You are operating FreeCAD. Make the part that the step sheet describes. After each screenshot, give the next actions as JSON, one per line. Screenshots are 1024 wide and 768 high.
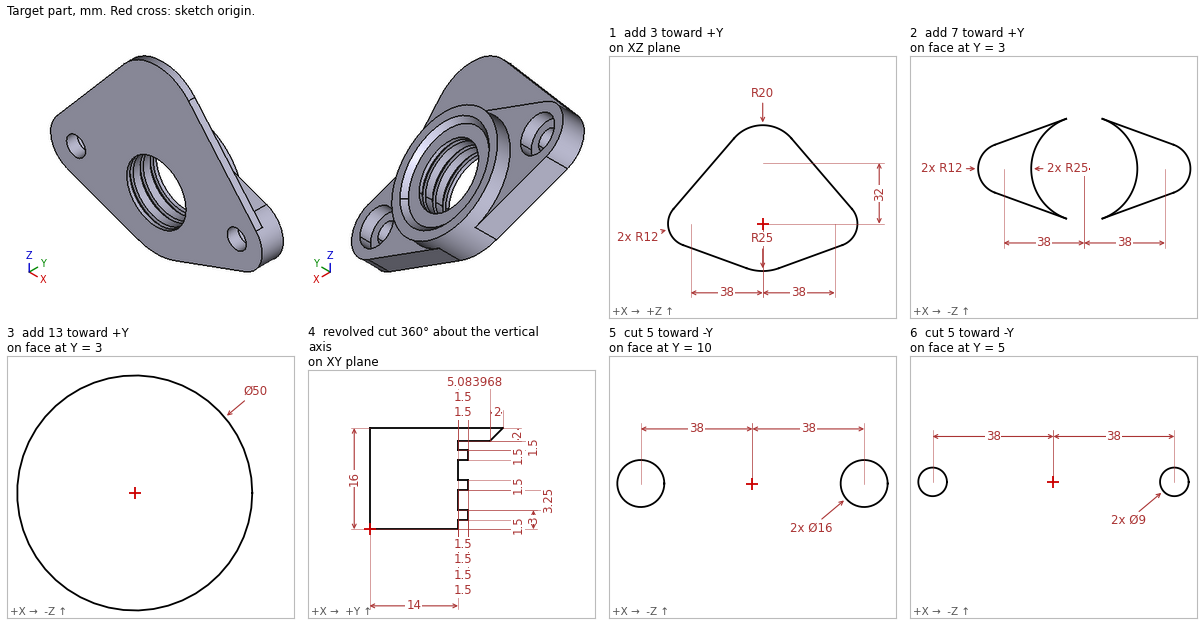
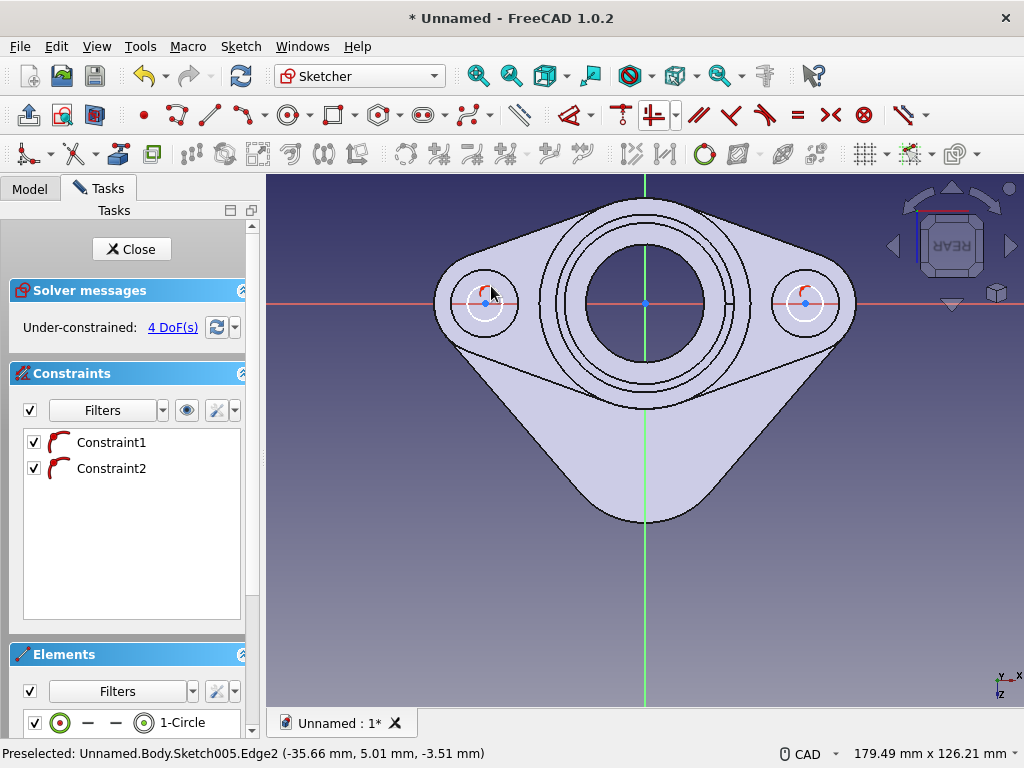
{"action": "left_click", "coordinate": [818, 291]}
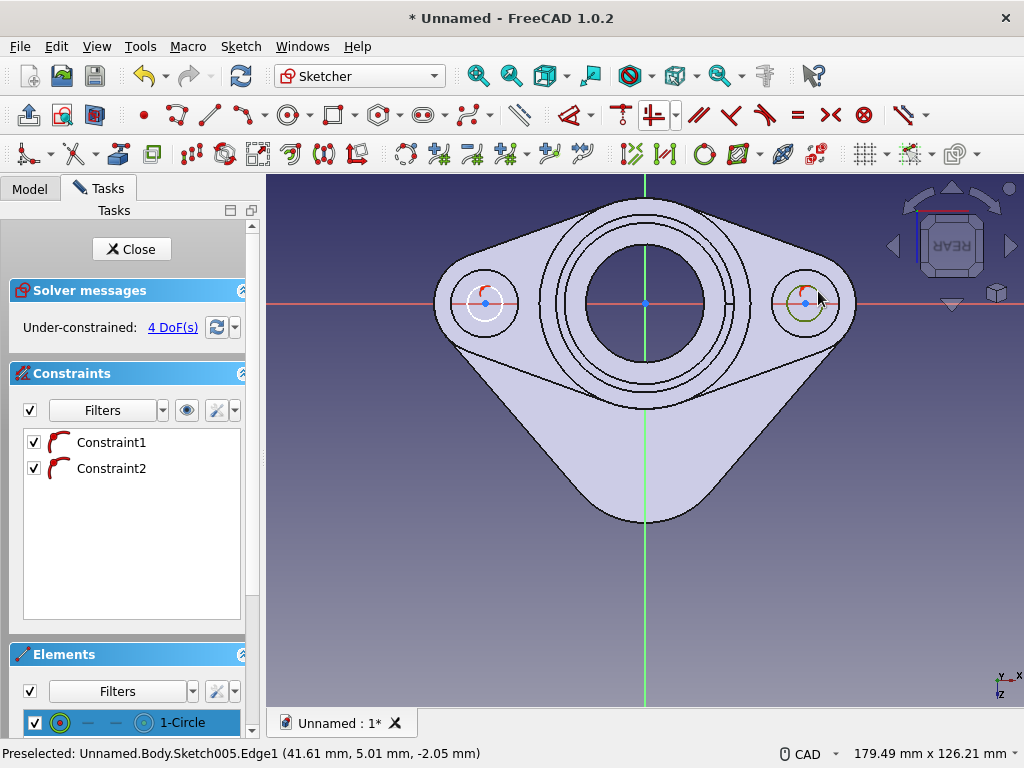
{"action": "left_click", "coordinate": [497, 291]}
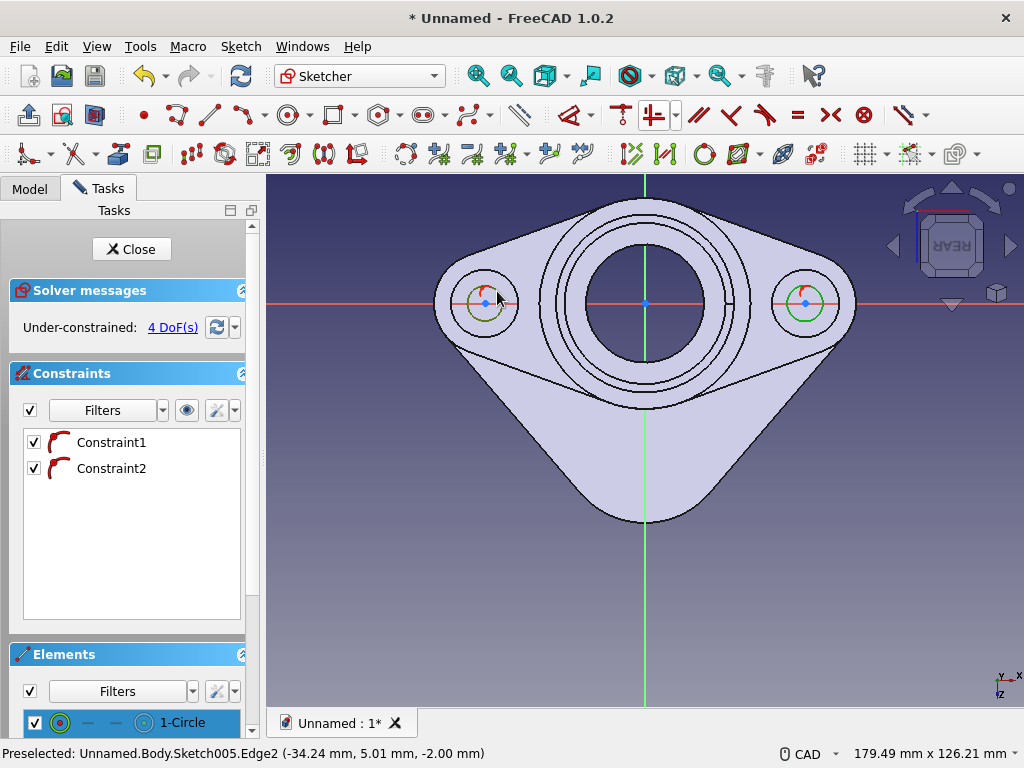
{"action": "left_click", "coordinate": [798, 116]}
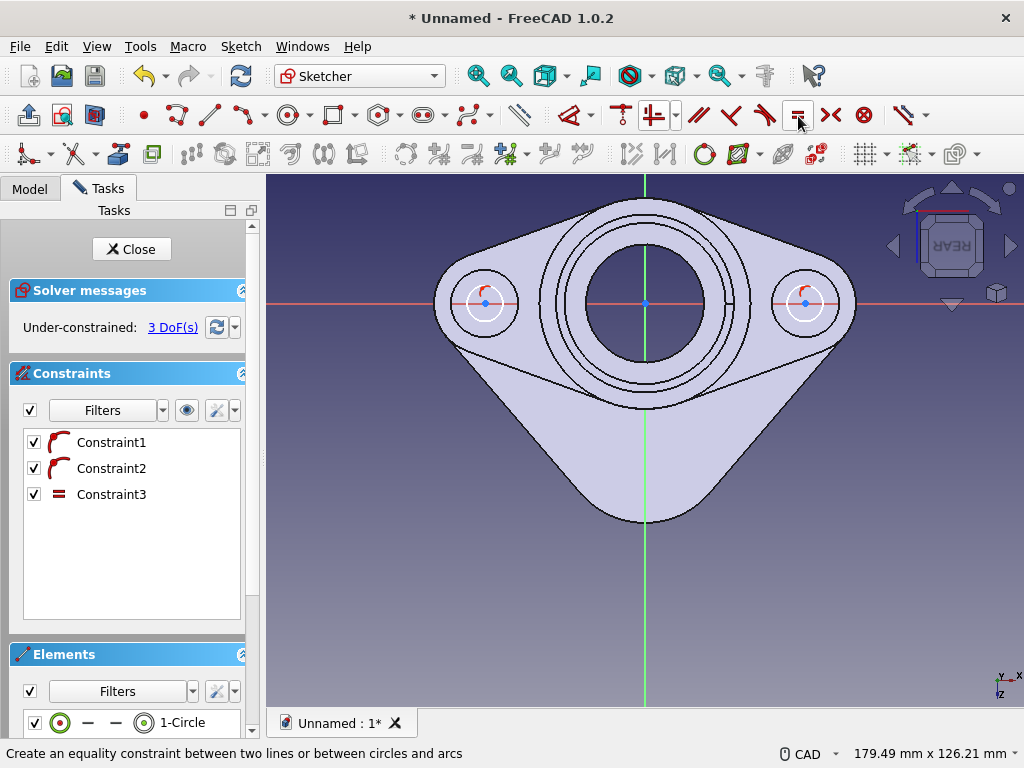
{"action": "left_click", "coordinate": [568, 116]}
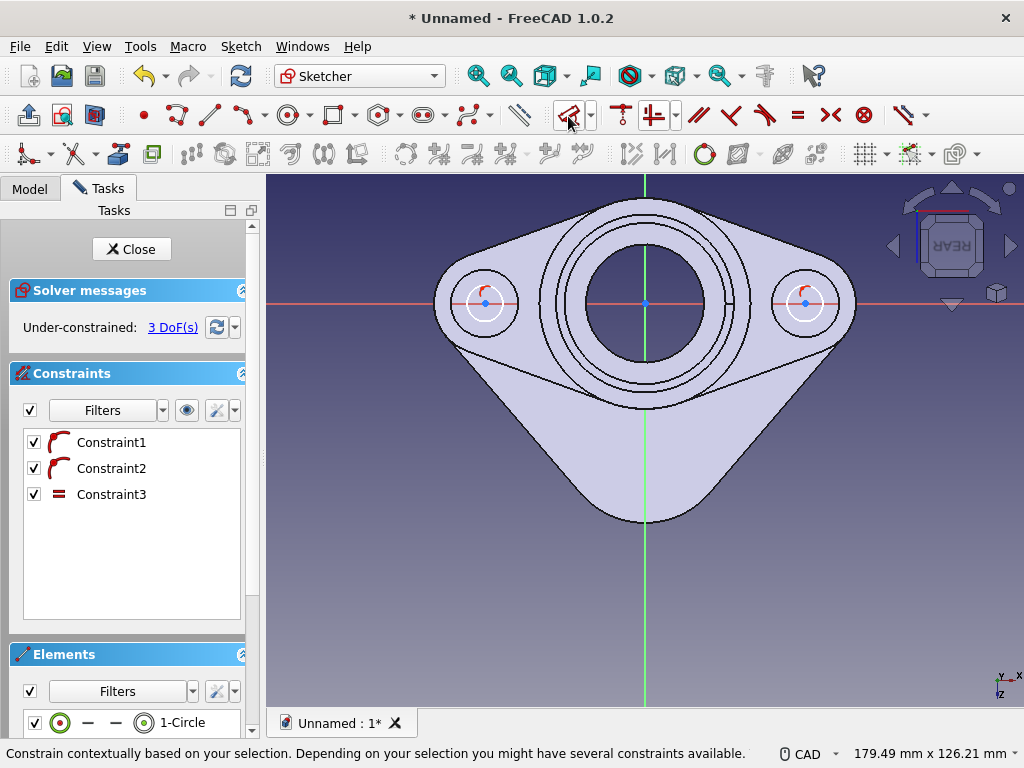
{"action": "left_click", "coordinate": [818, 291]}
{"action": "left_click", "coordinate": [841, 269]}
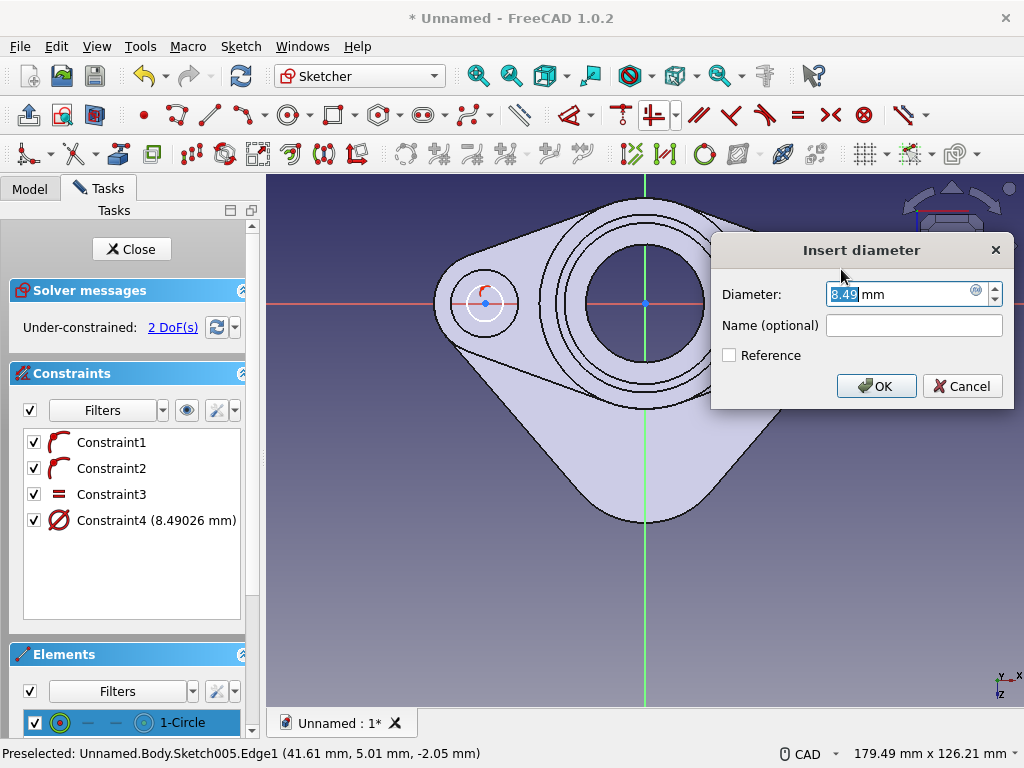
{"action": "type", "text": "9"}
{"action": "key", "text": "Return"}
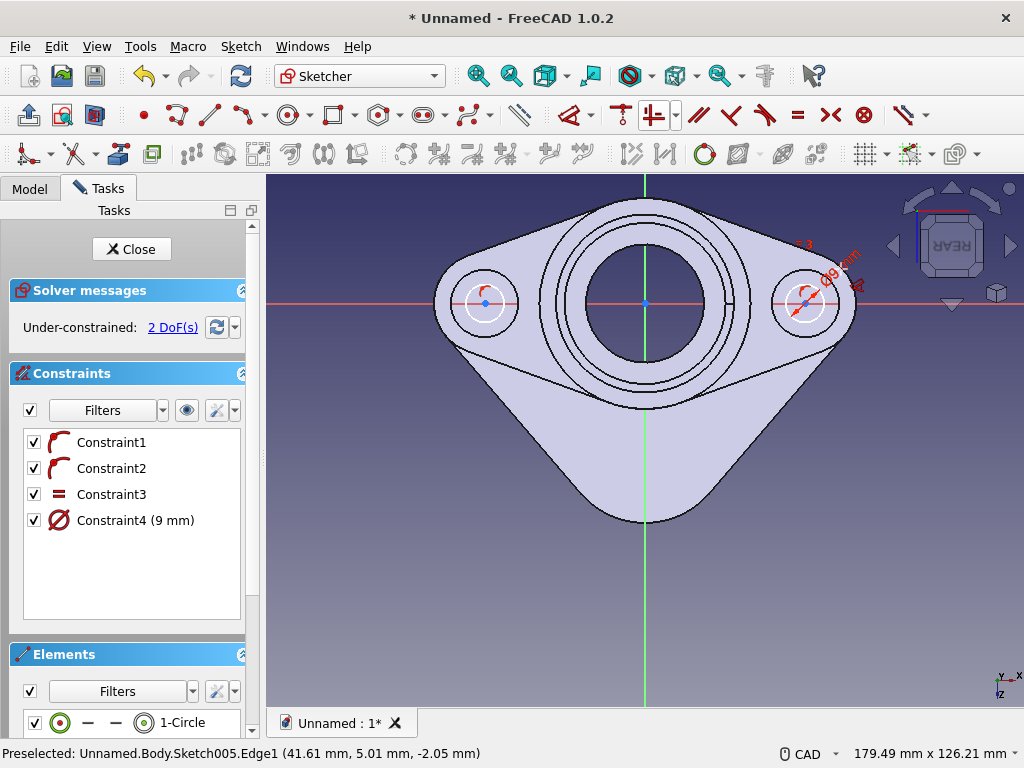
{"action": "left_click", "coordinate": [805, 304]}
{"action": "left_click", "coordinate": [725, 338]}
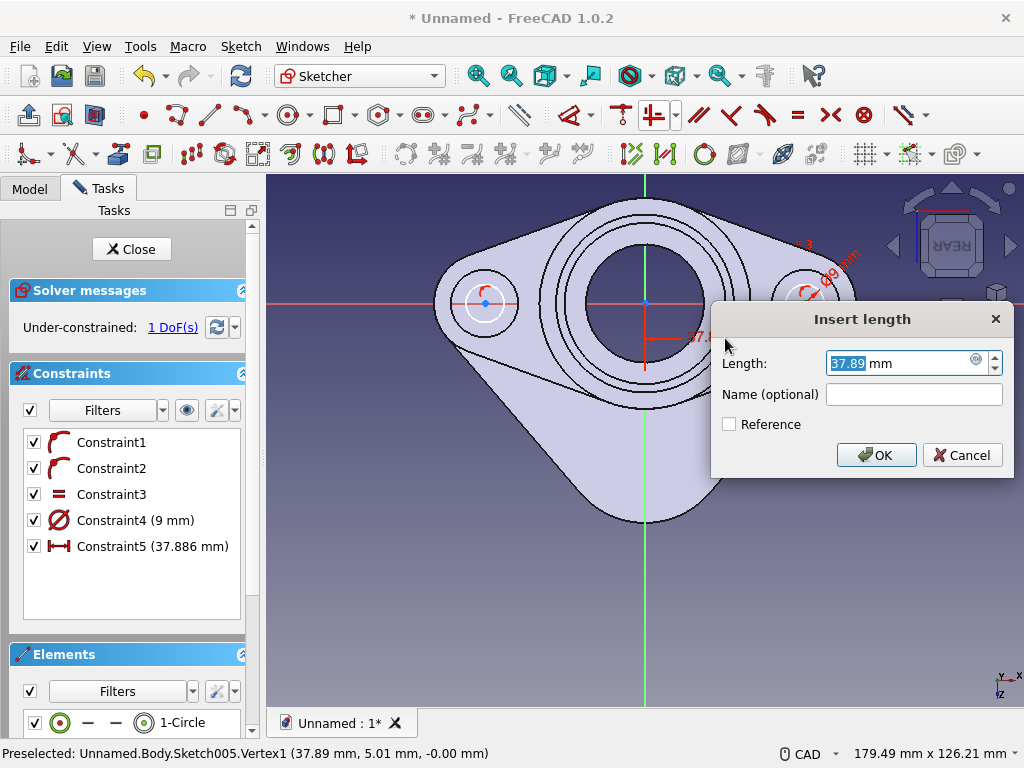
{"action": "type", "text": "38"}
{"action": "key", "text": "Return"}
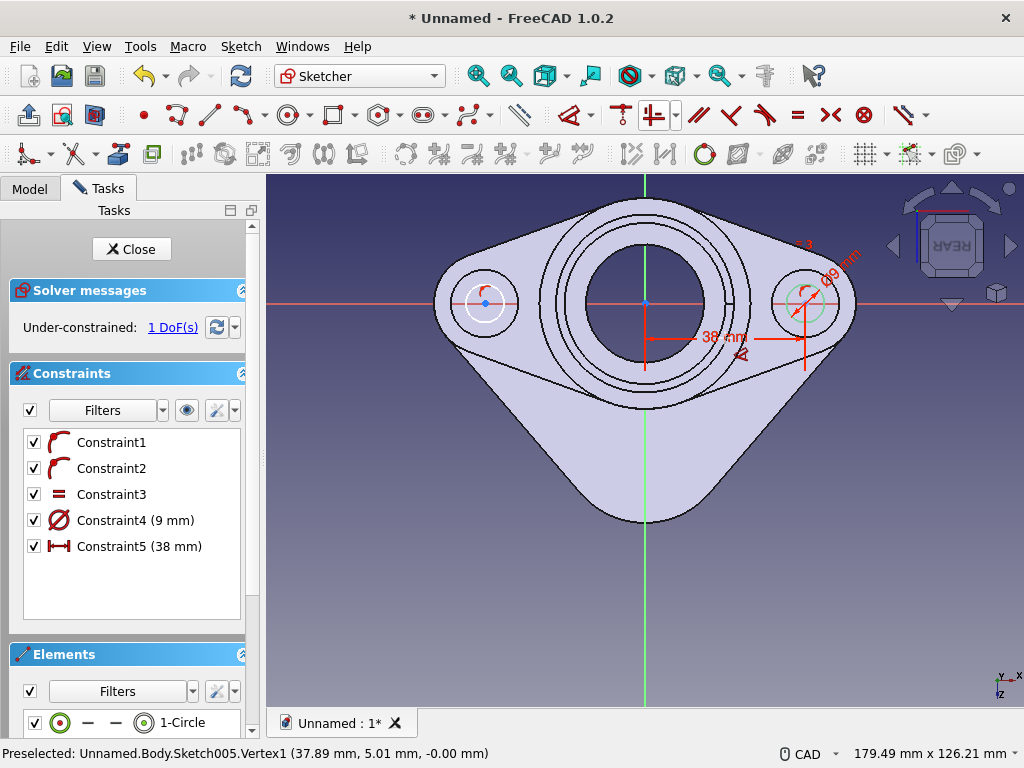
{"action": "left_click", "coordinate": [485, 304]}
{"action": "left_click", "coordinate": [565, 338]}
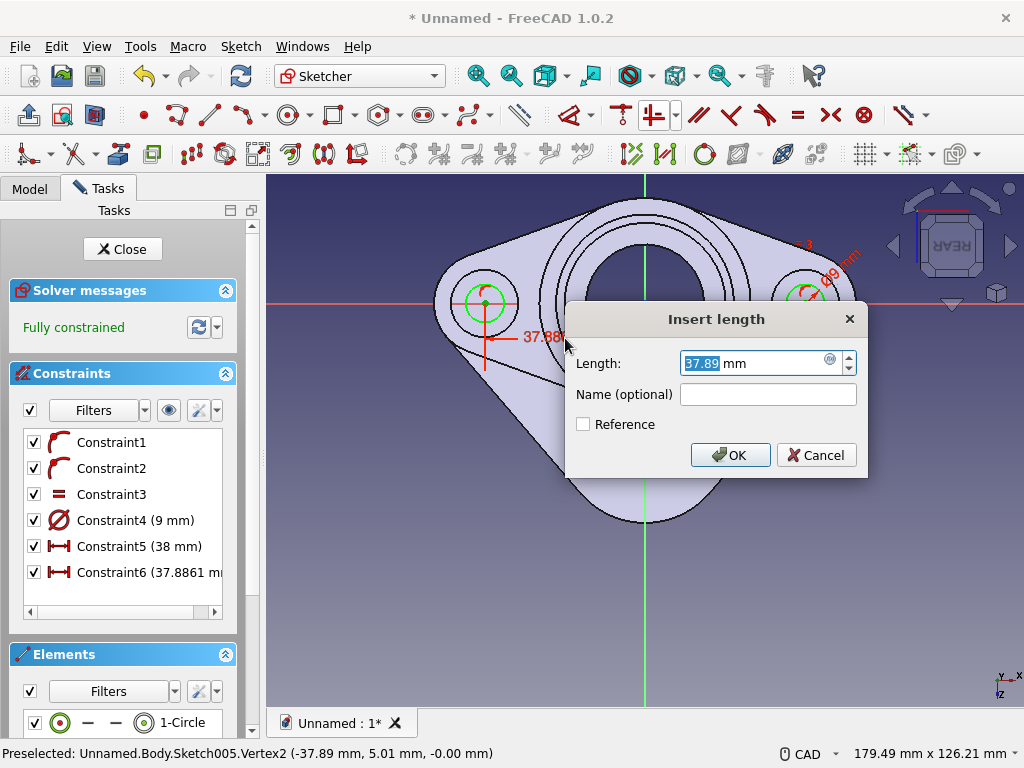
{"action": "type", "text": "38"}
{"action": "key", "text": "Return"}
{"action": "key", "text": "Escape"}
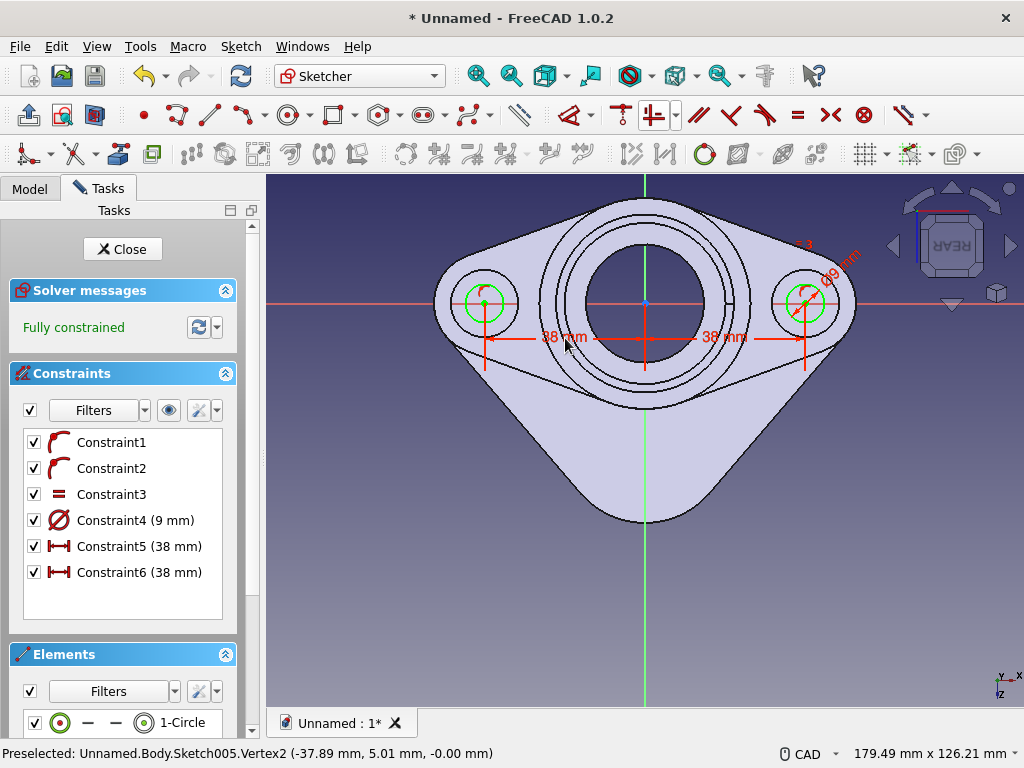
{"action": "left_click", "coordinate": [123, 249]}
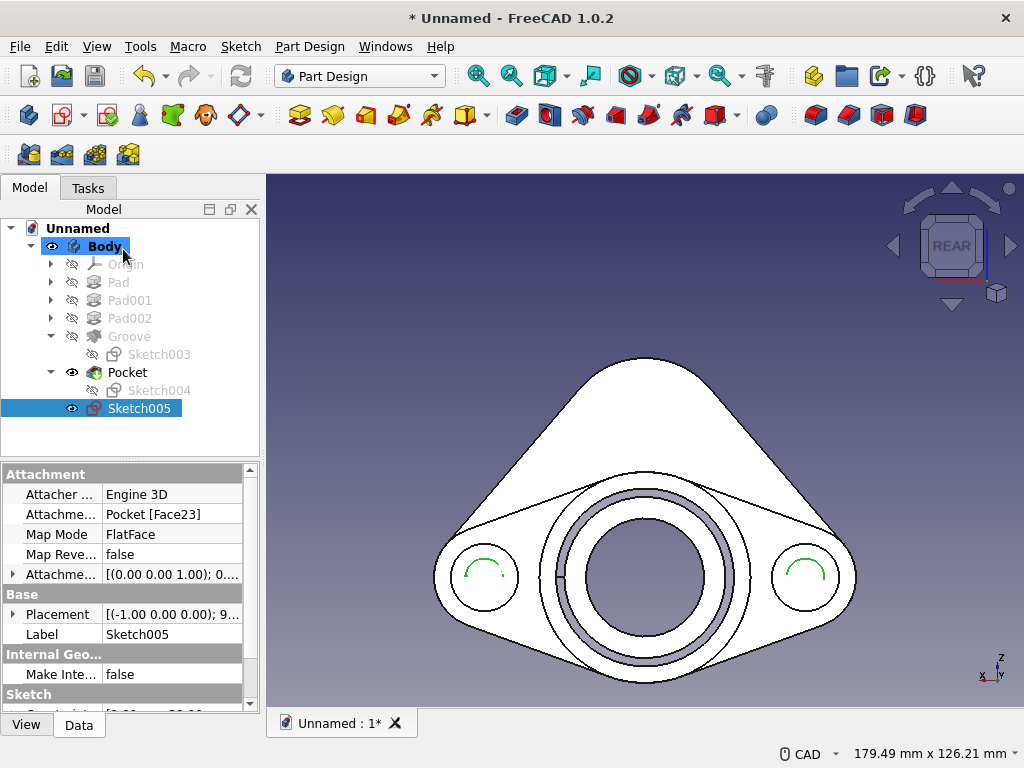
{"action": "left_click", "coordinate": [517, 116]}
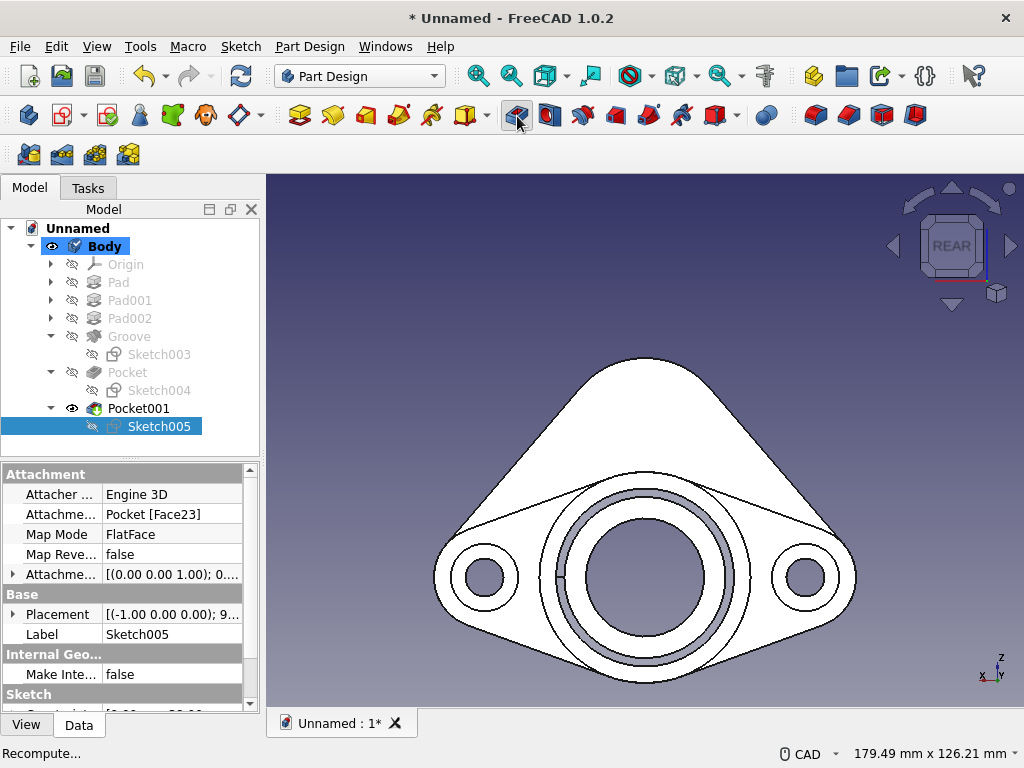
{"action": "type", "text": "5"}
{"action": "key", "text": "Tab"}